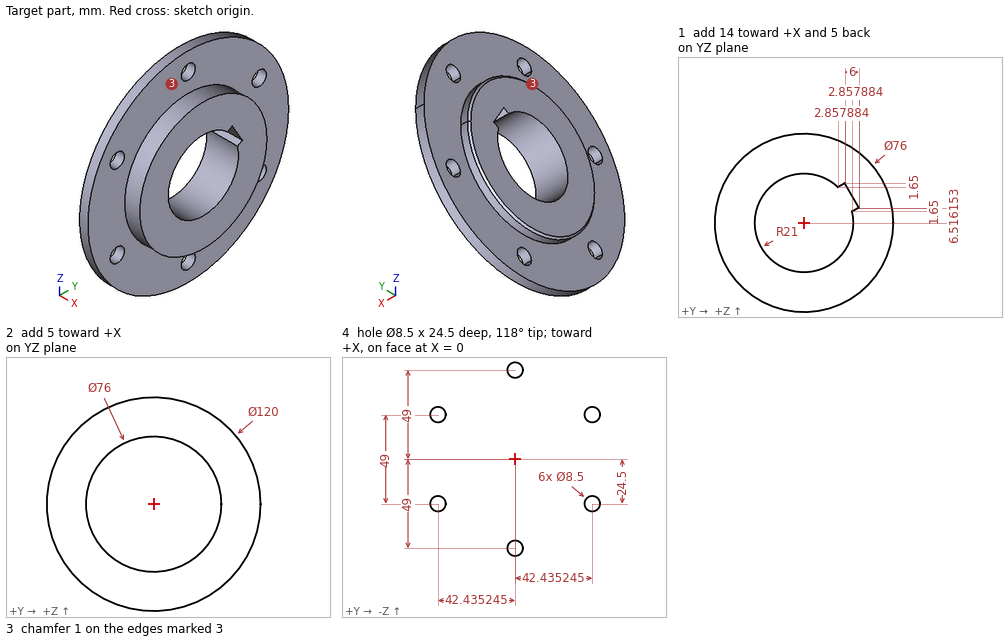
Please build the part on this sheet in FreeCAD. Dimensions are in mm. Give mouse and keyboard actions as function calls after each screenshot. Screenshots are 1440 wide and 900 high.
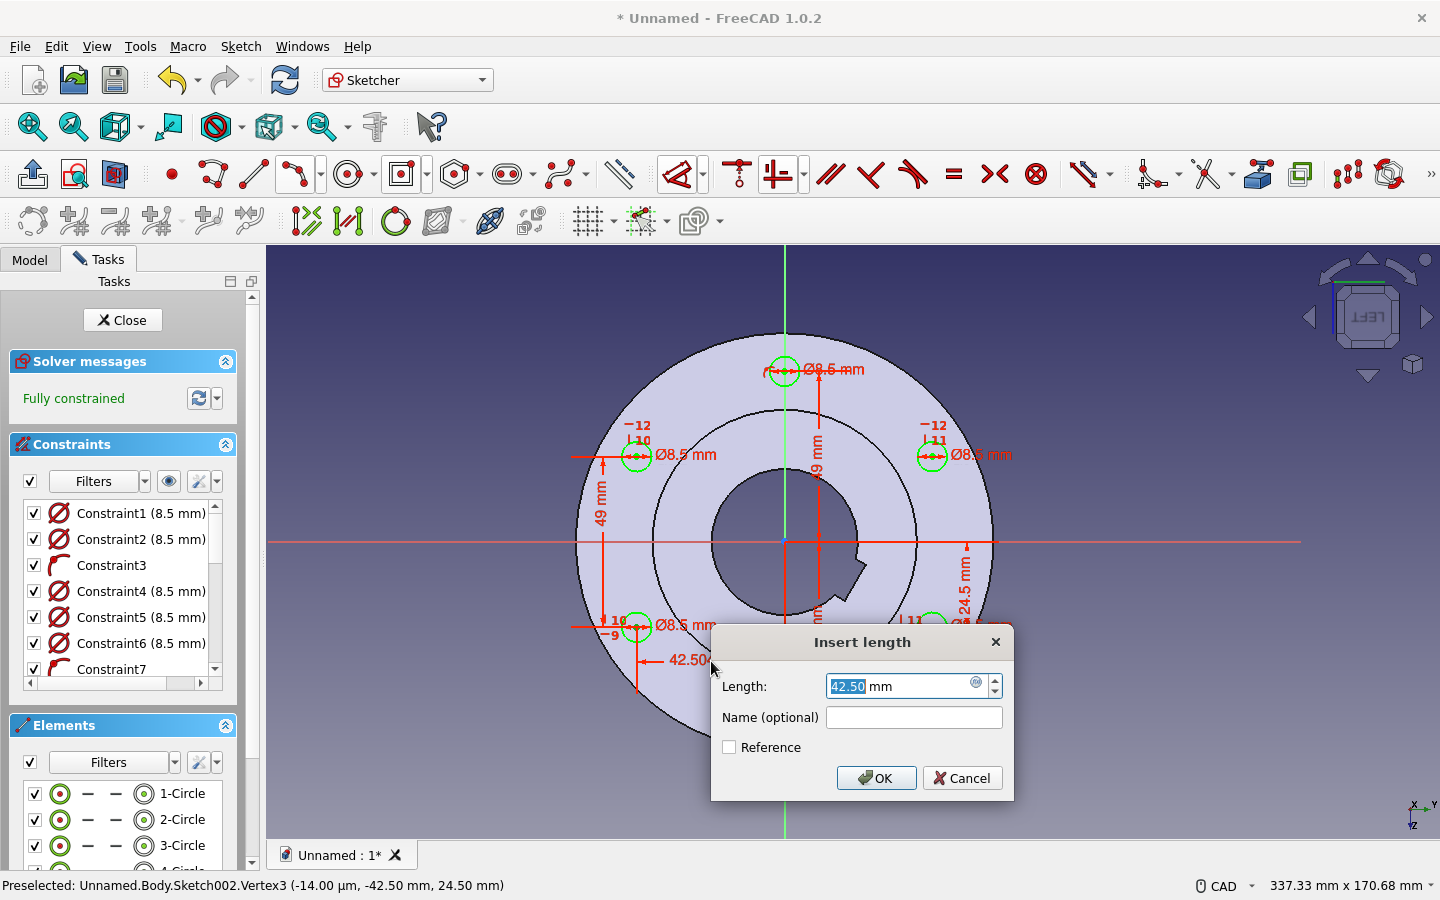
text(42.435245)
key(Return)
key(Escape)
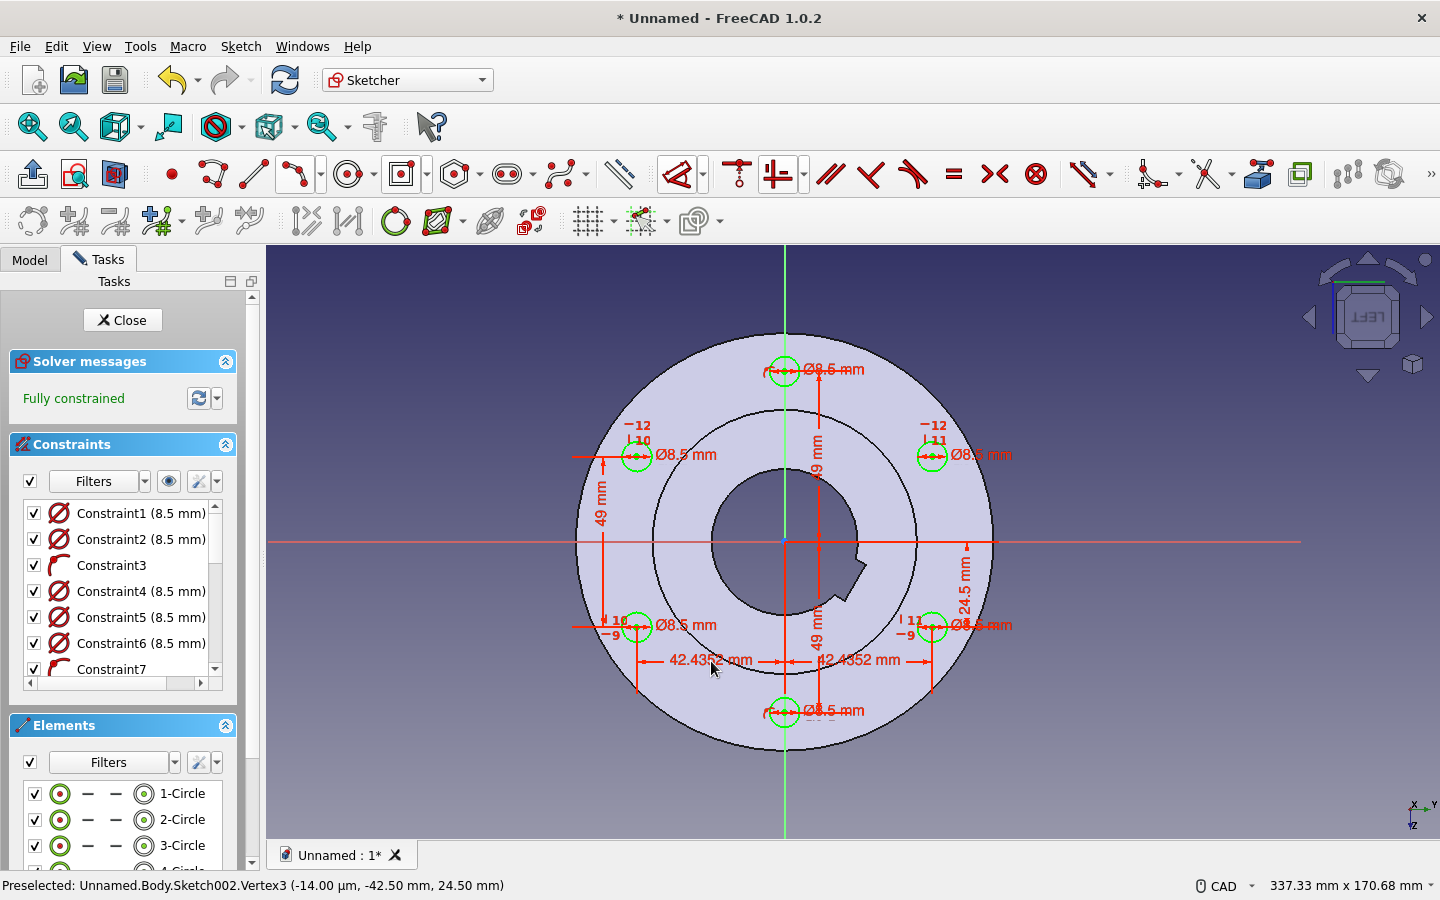
click(123, 320)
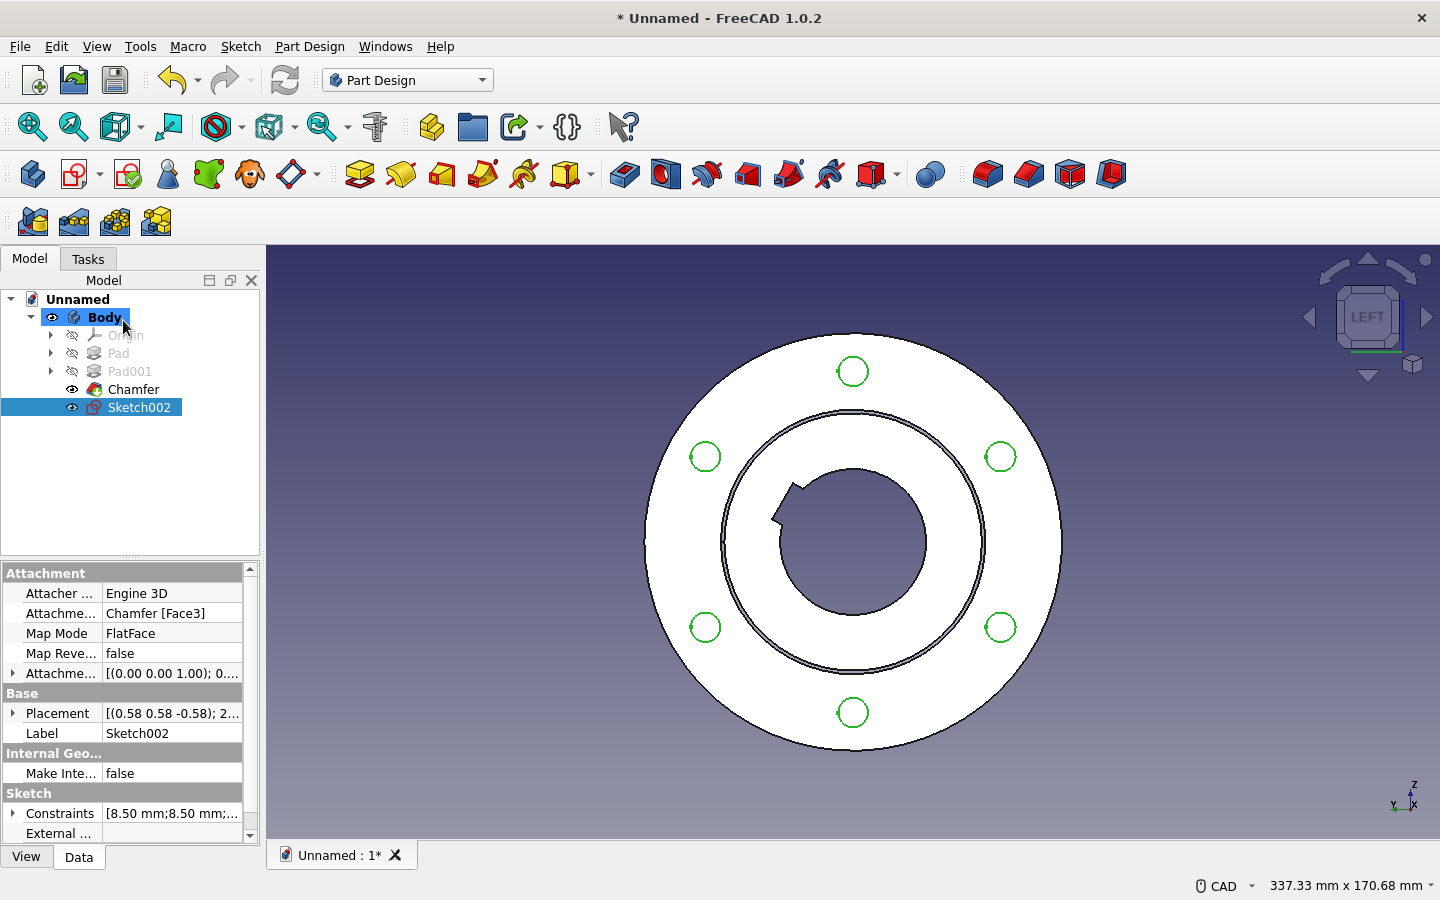
click(666, 174)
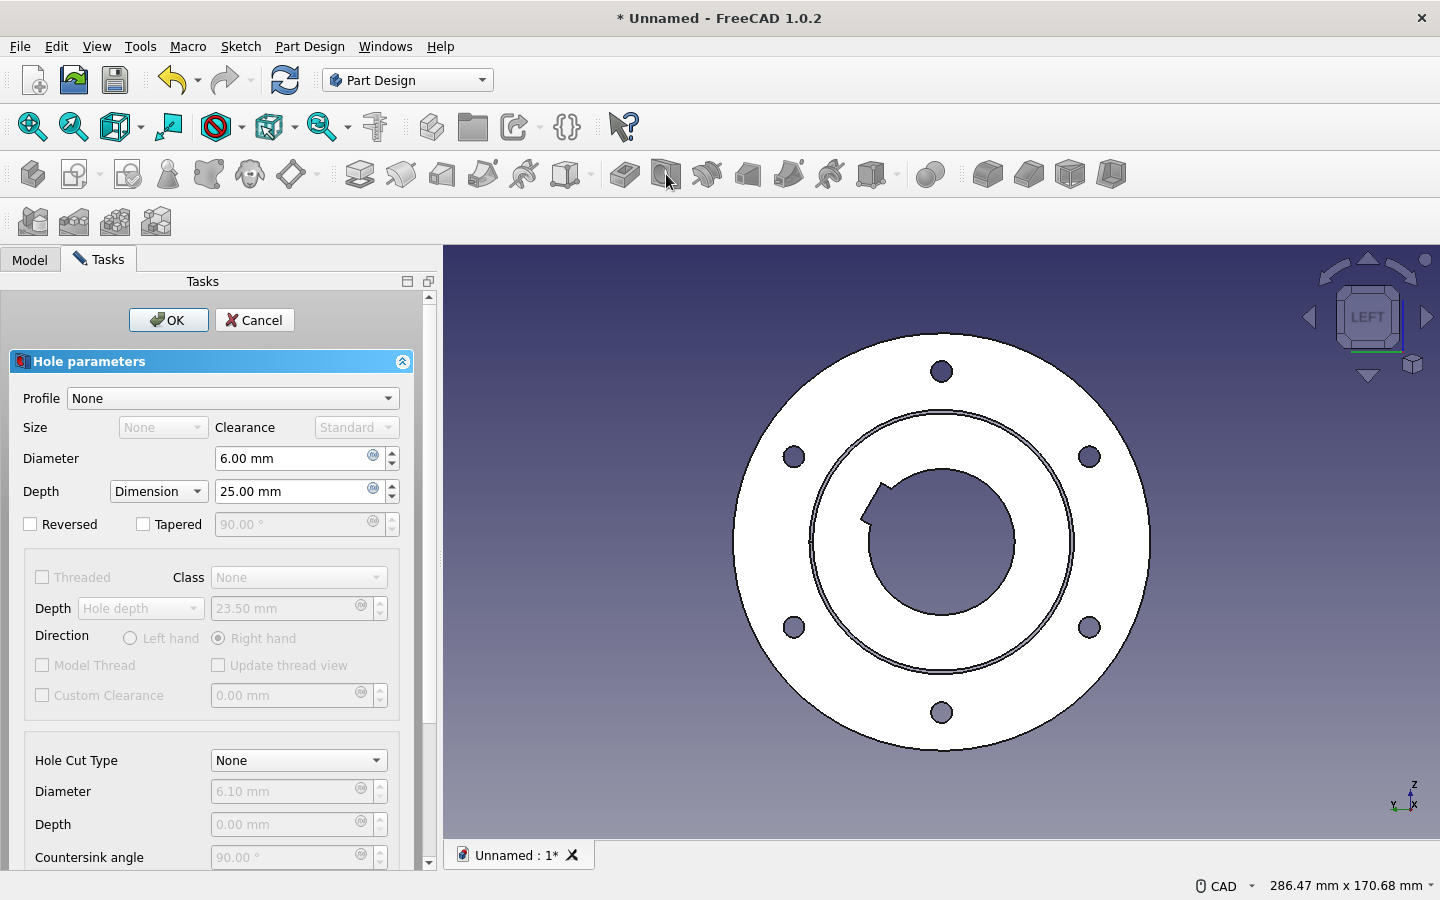
triple_click(300, 458)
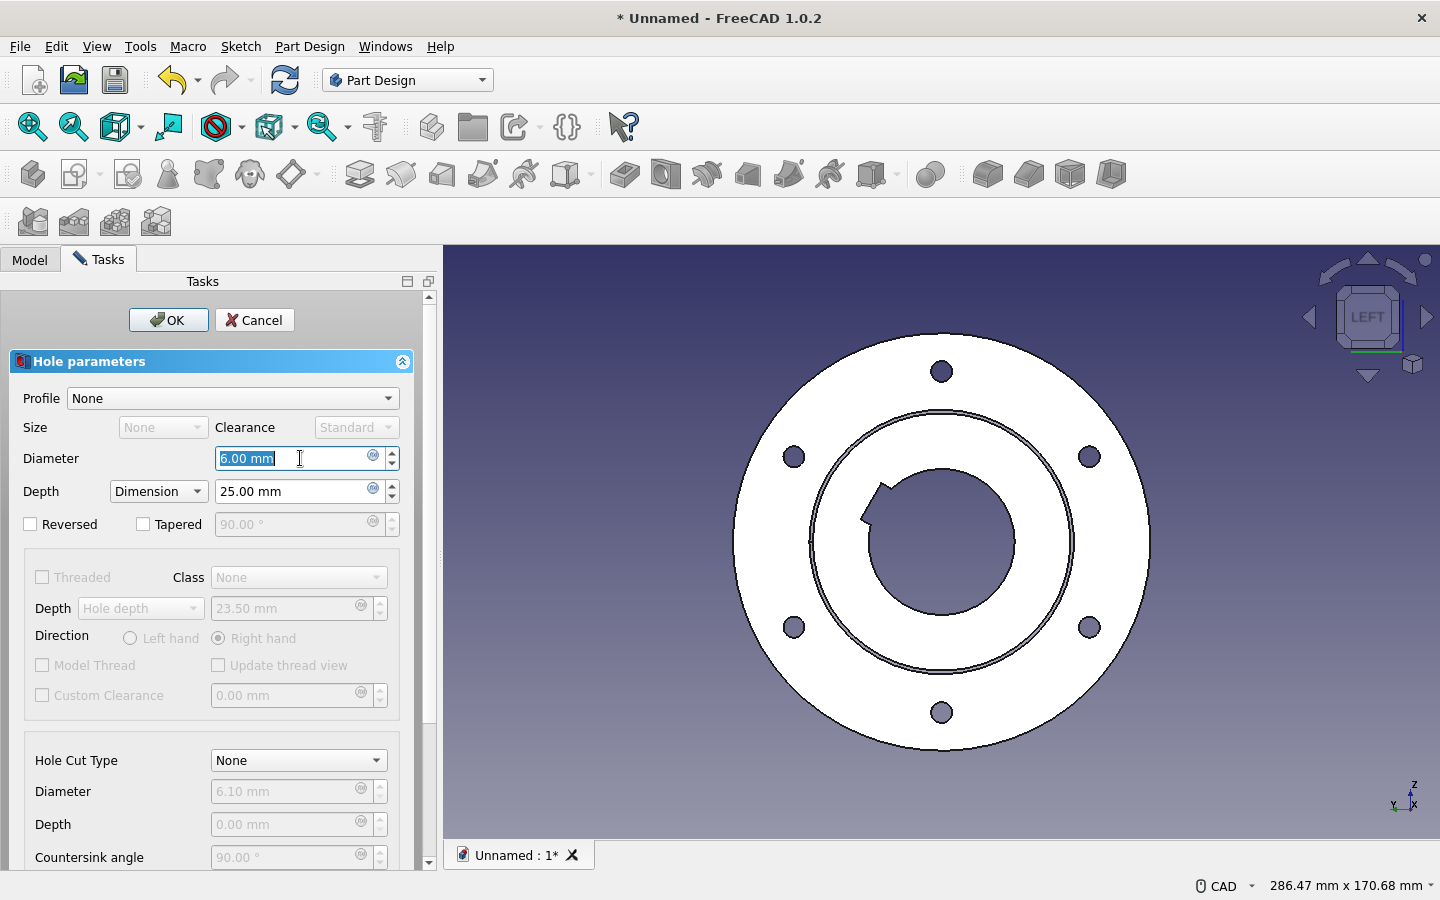
text(8.5)
key(Tab)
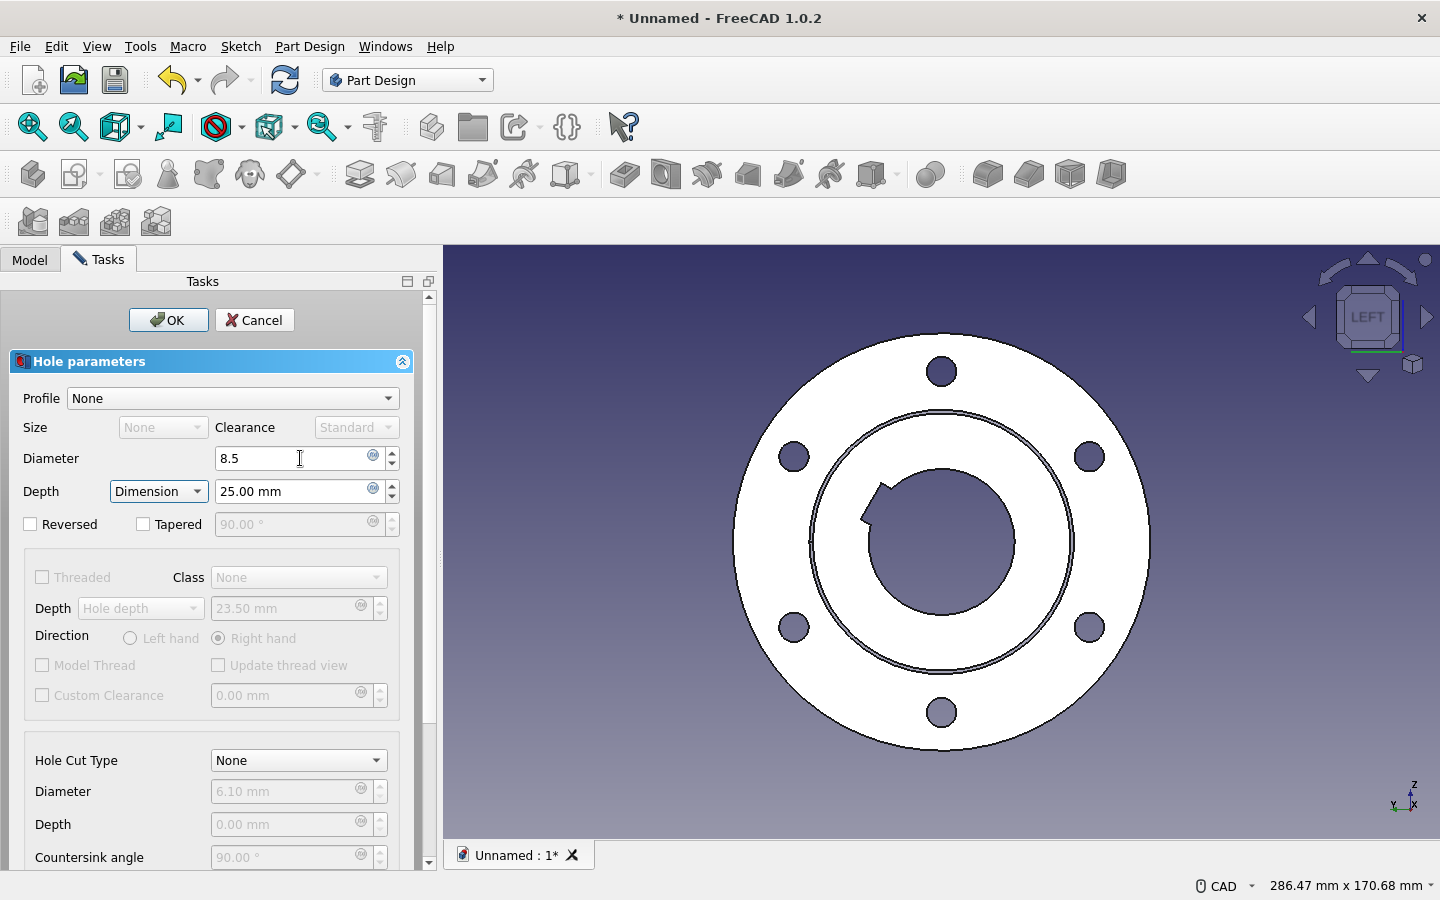
triple_click(300, 492)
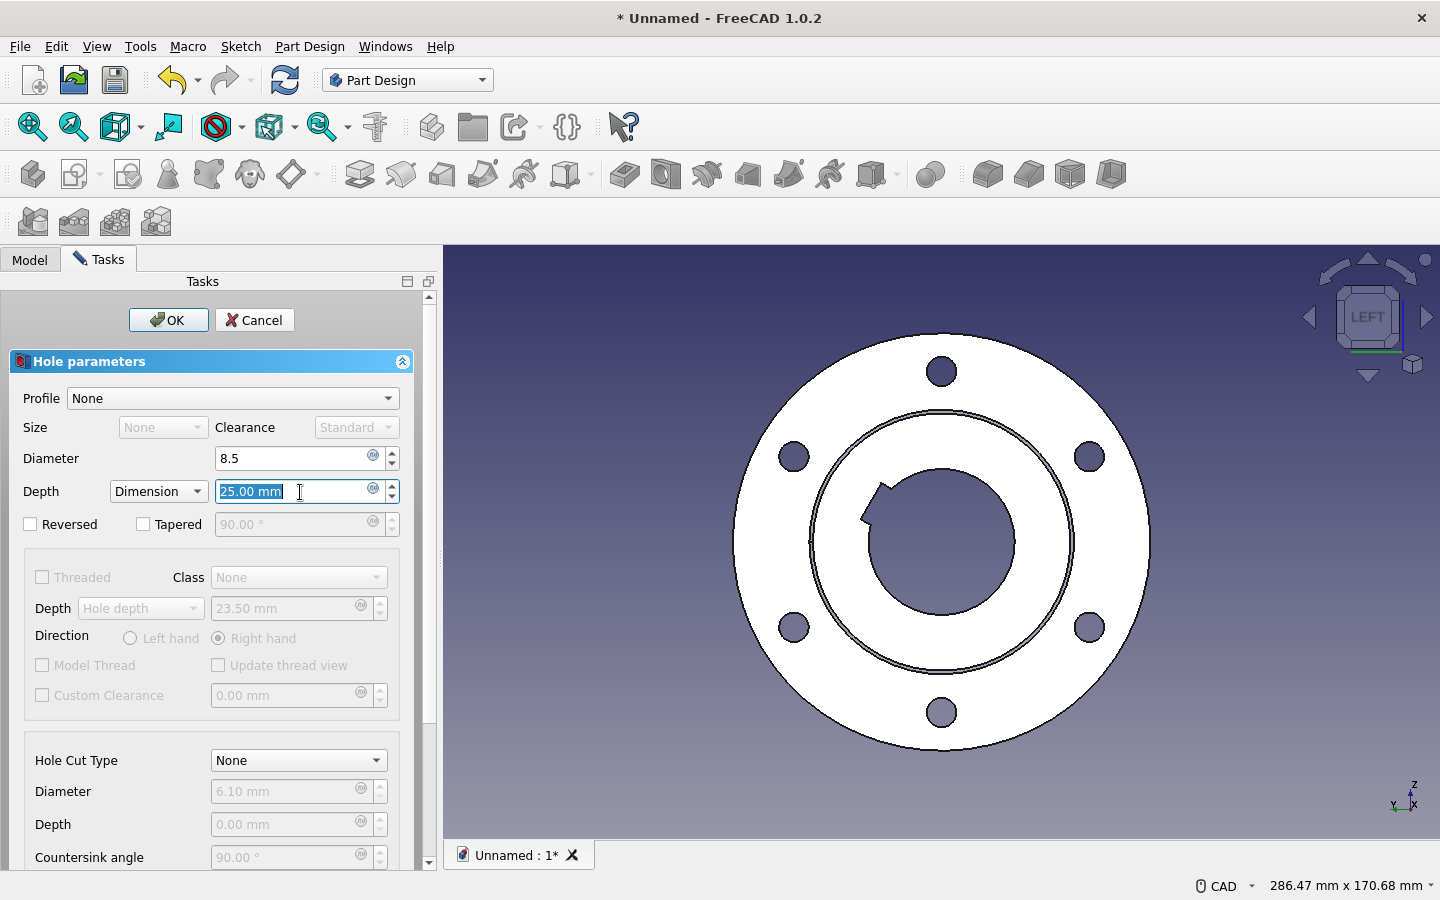
text(24.5)
key(Tab)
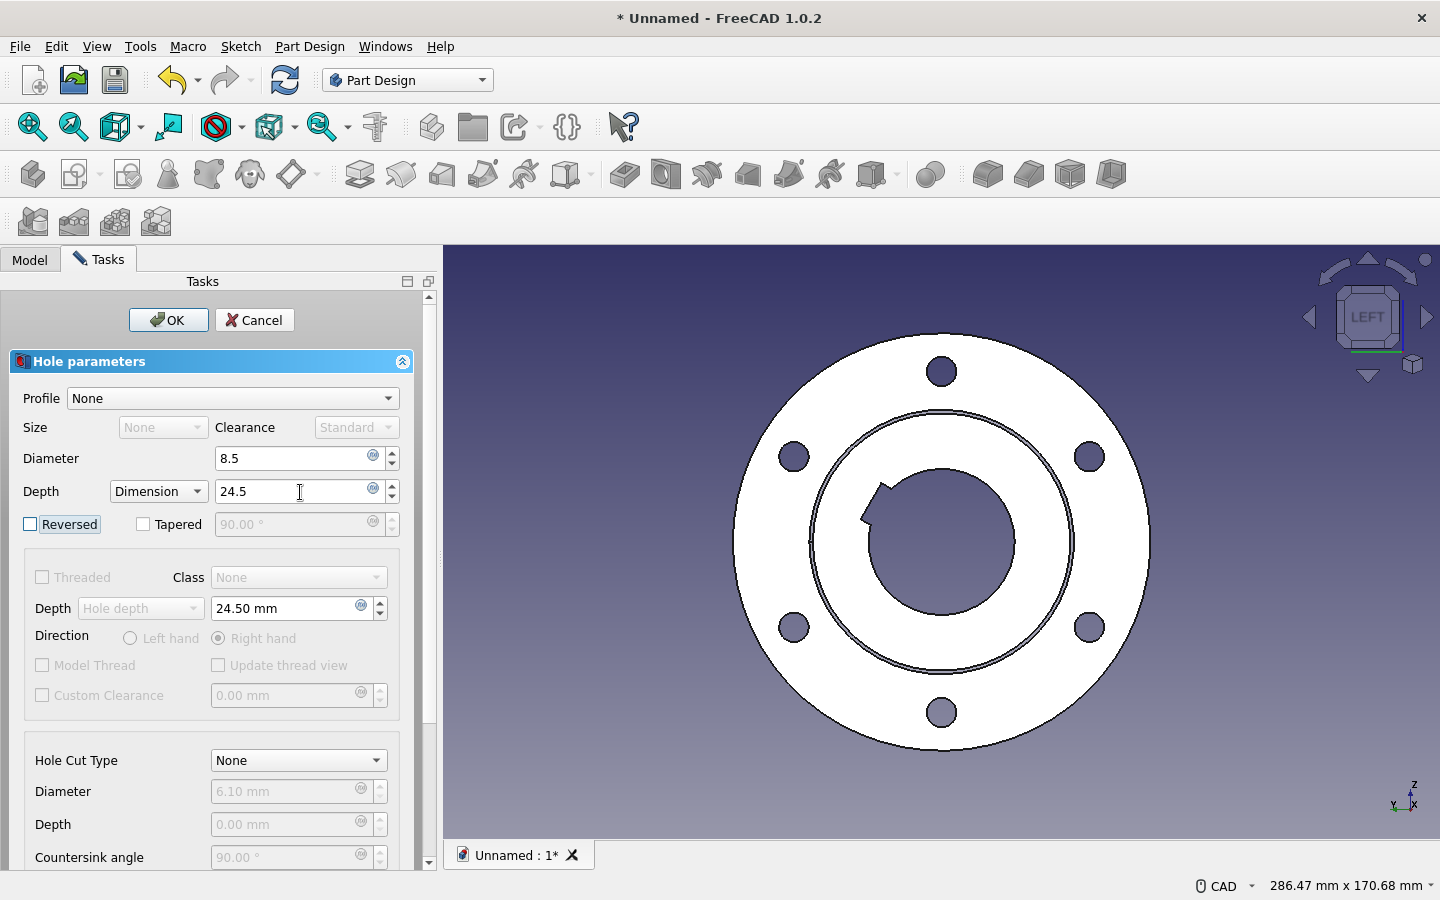
click(169, 320)